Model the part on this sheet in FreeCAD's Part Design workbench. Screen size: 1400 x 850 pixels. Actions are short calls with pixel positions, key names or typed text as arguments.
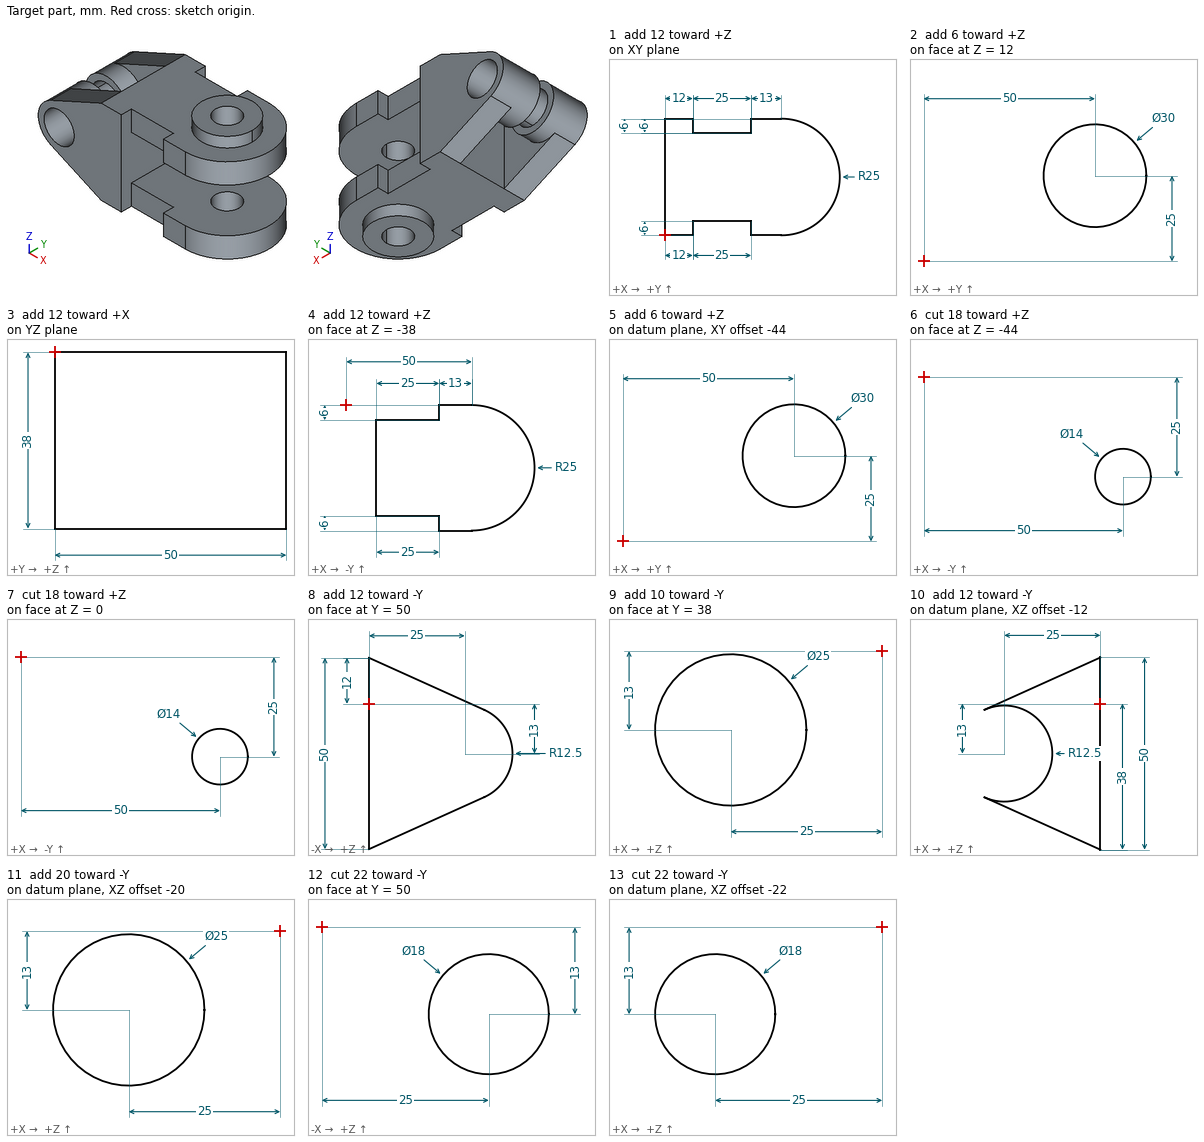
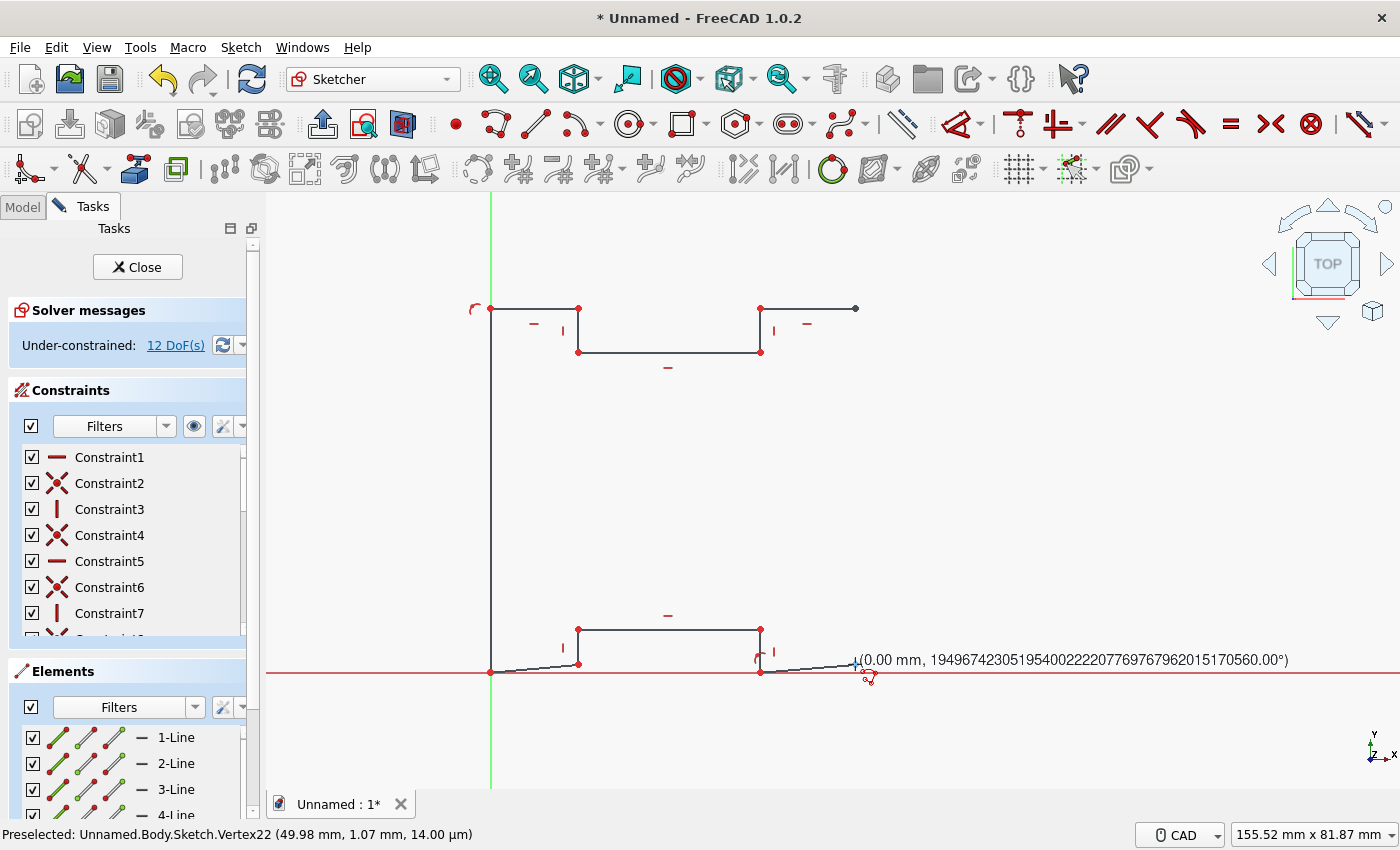
click(602, 124)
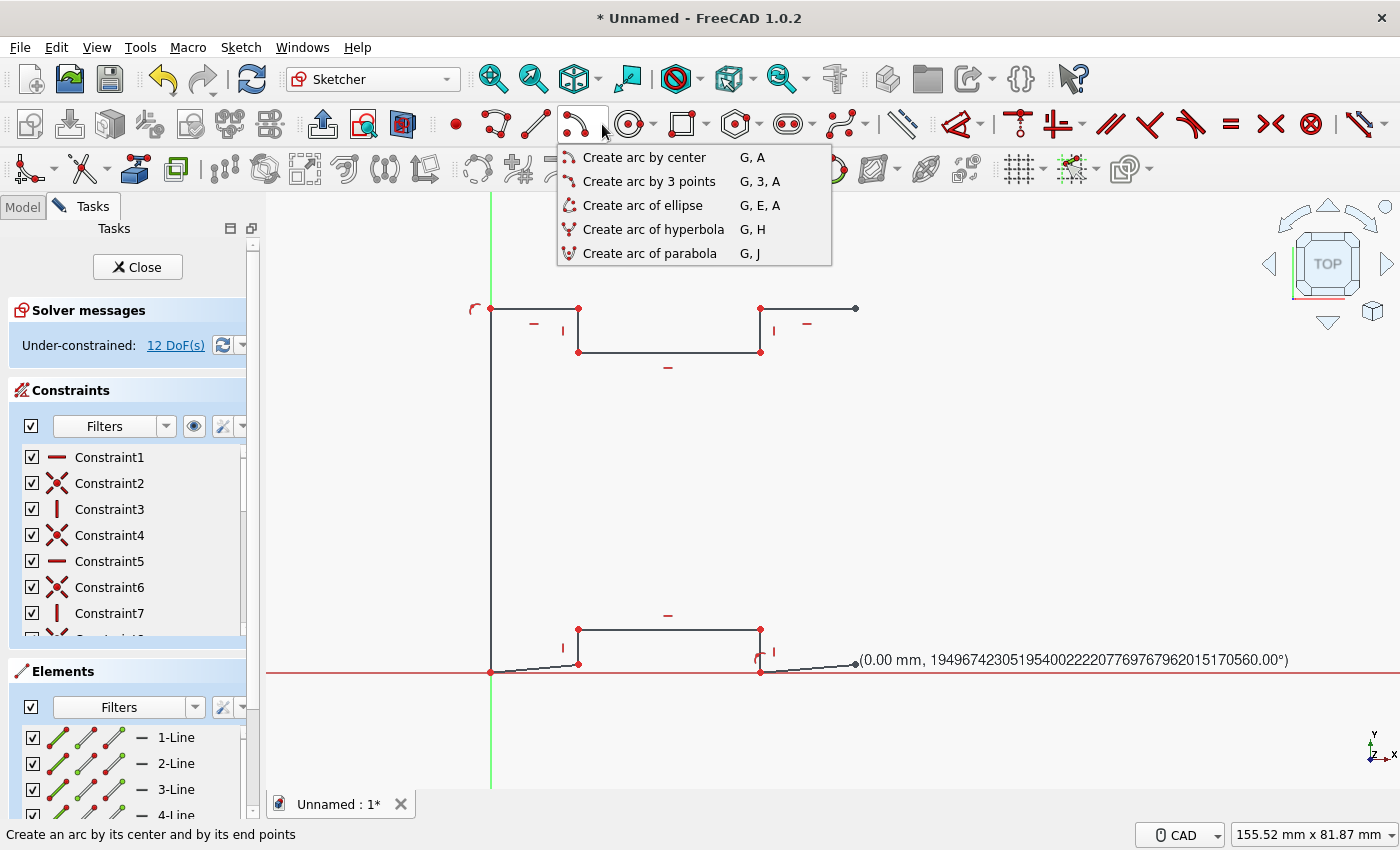
click(694, 181)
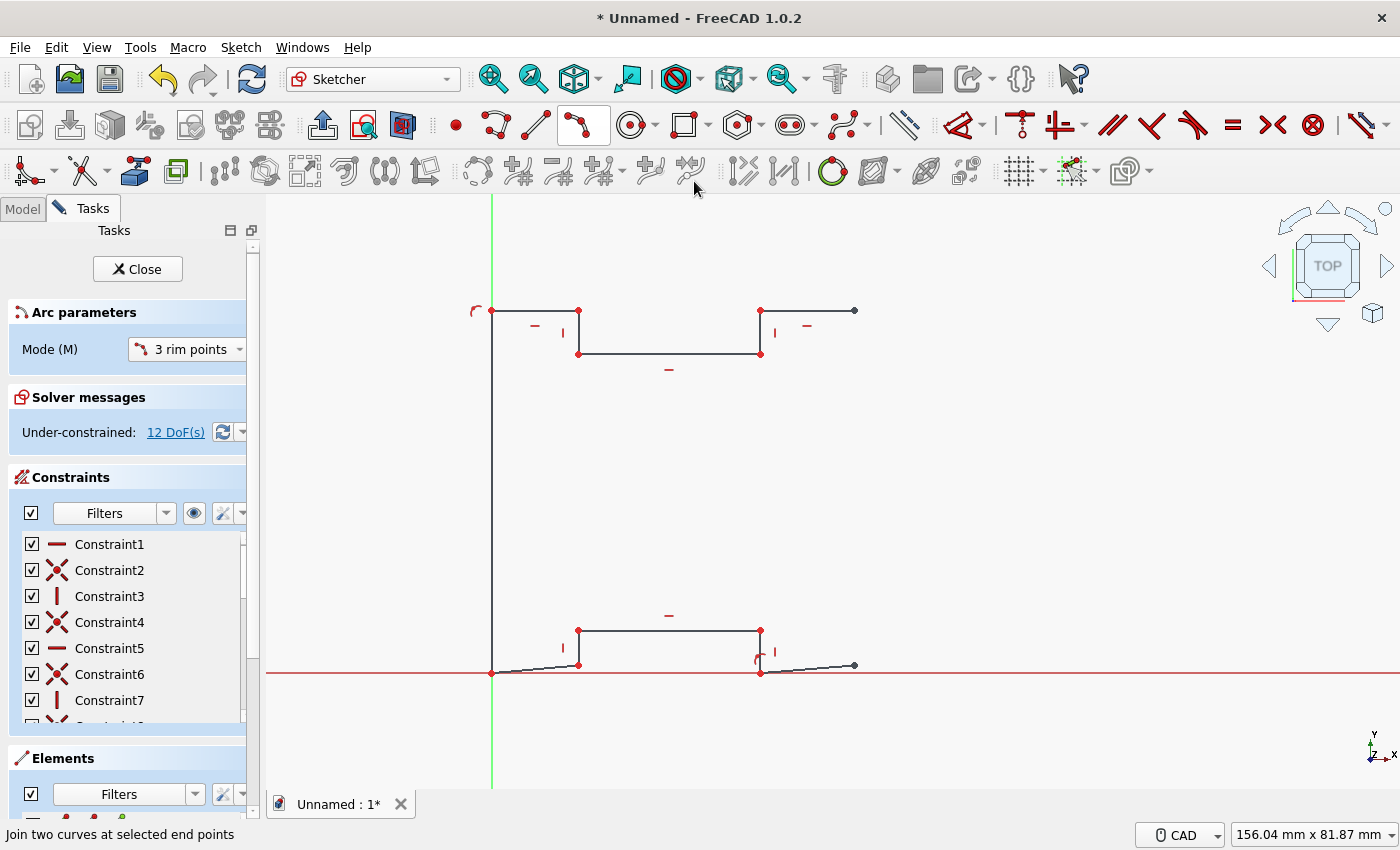
click(855, 665)
click(855, 311)
click(1037, 491)
key(Escape)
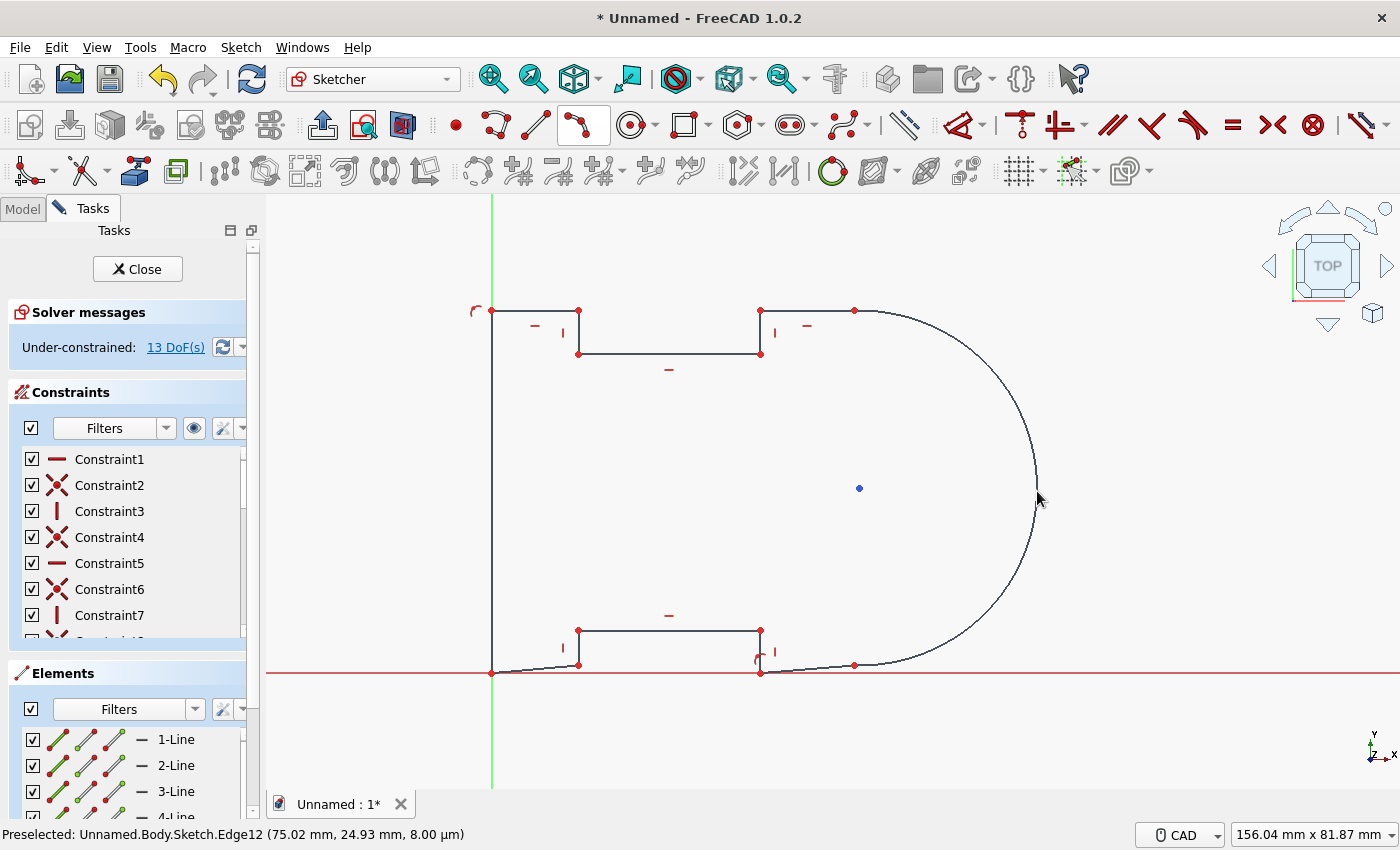
click(827, 311)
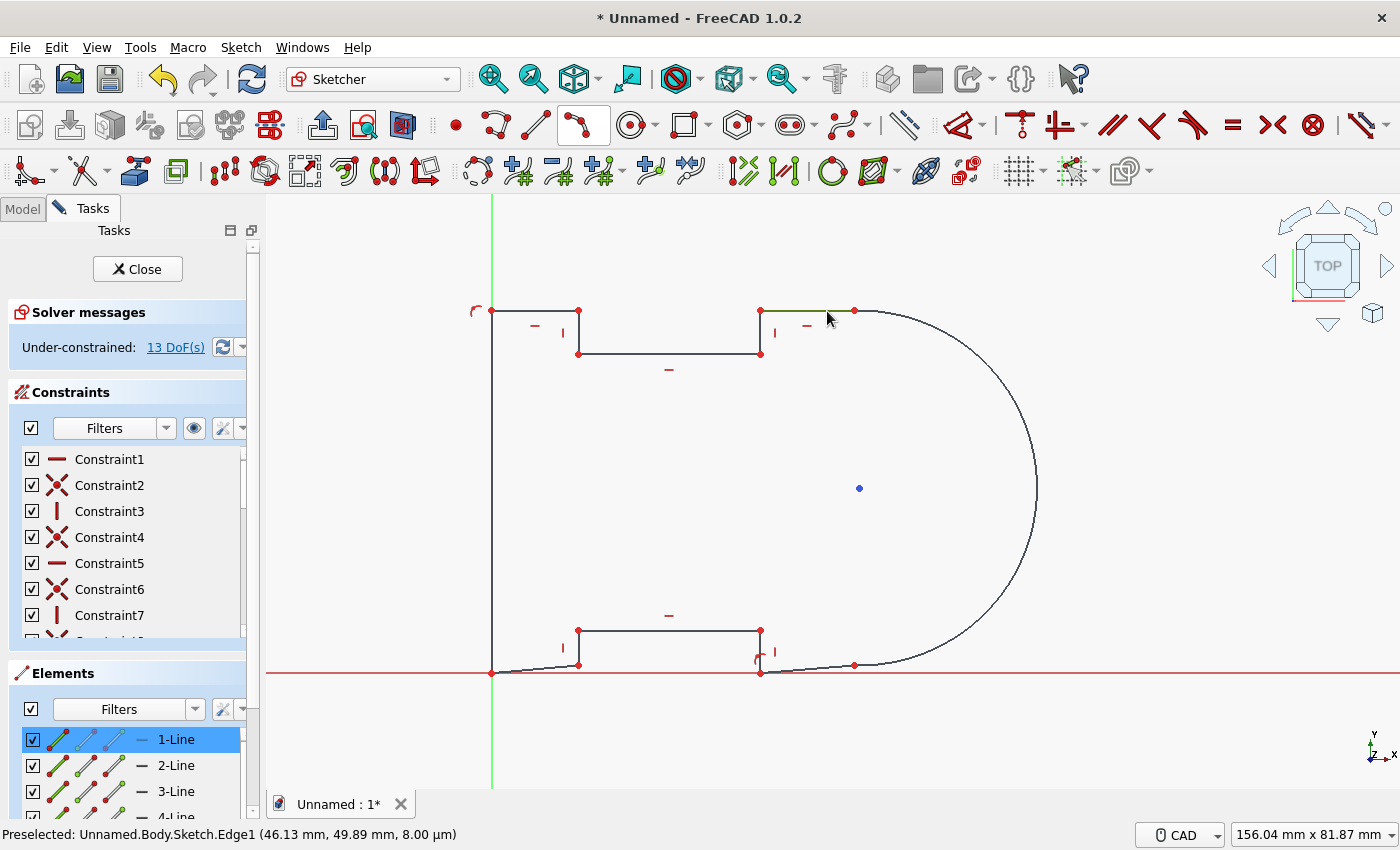
click(1002, 594)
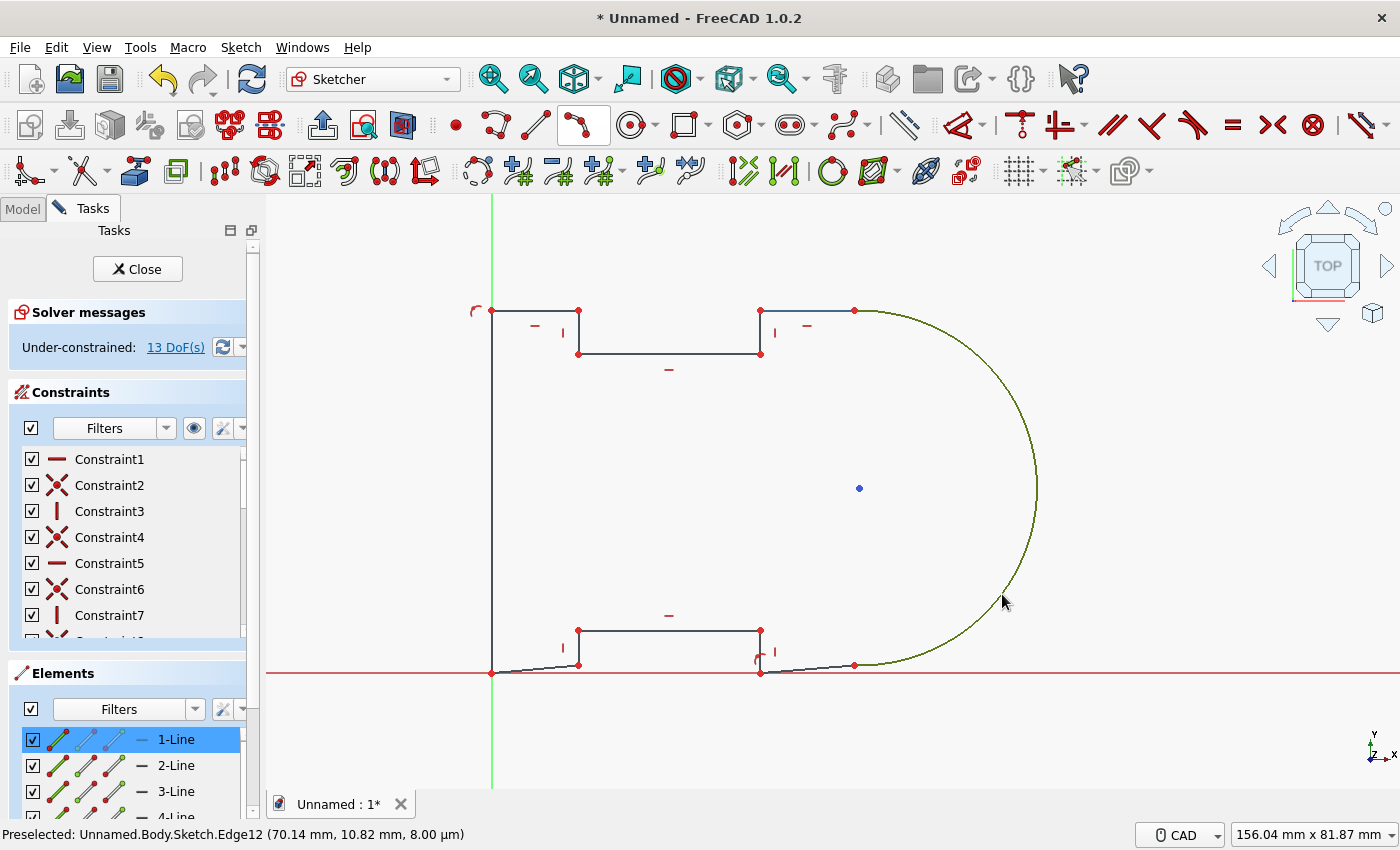
click(1194, 126)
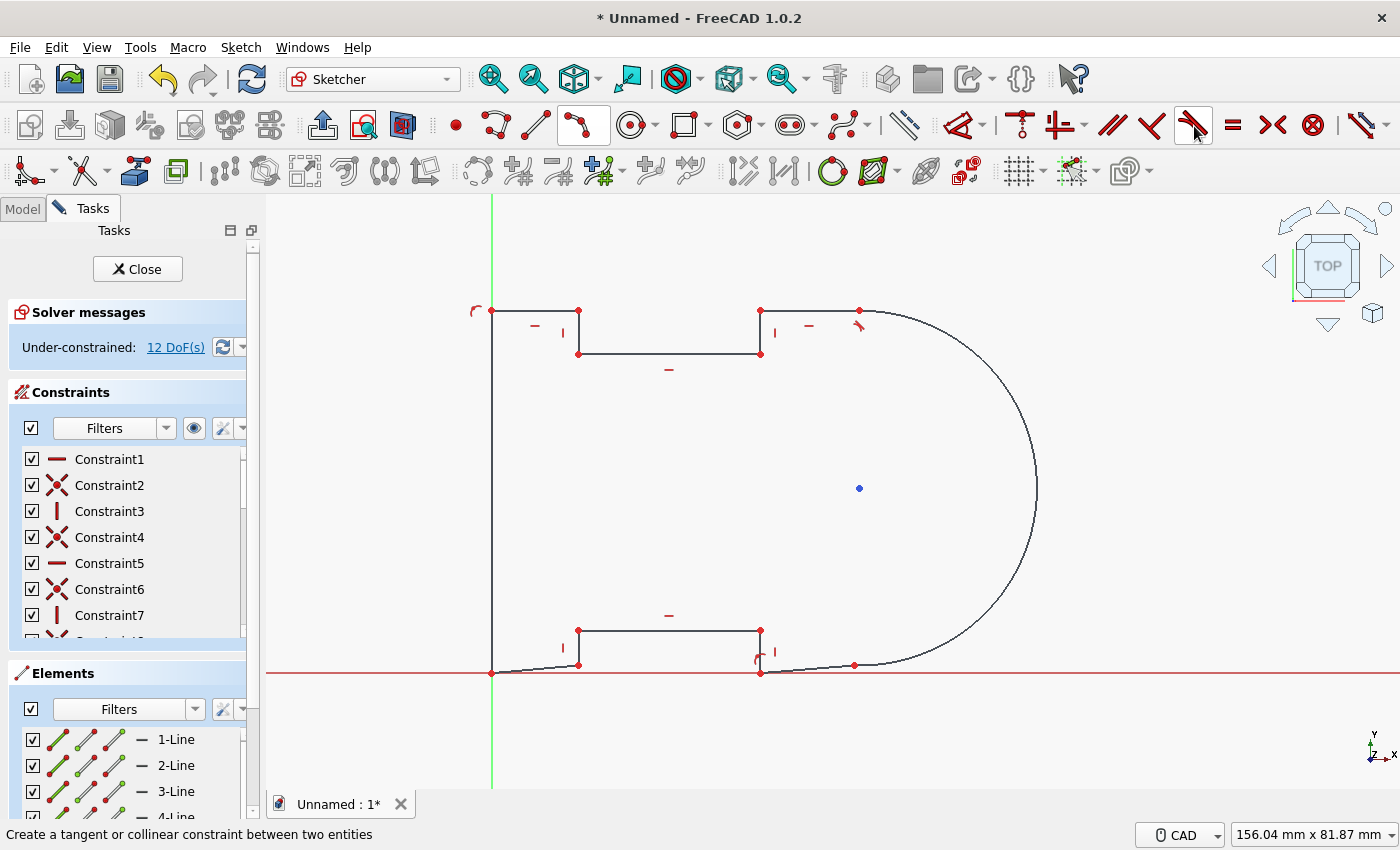
click(789, 671)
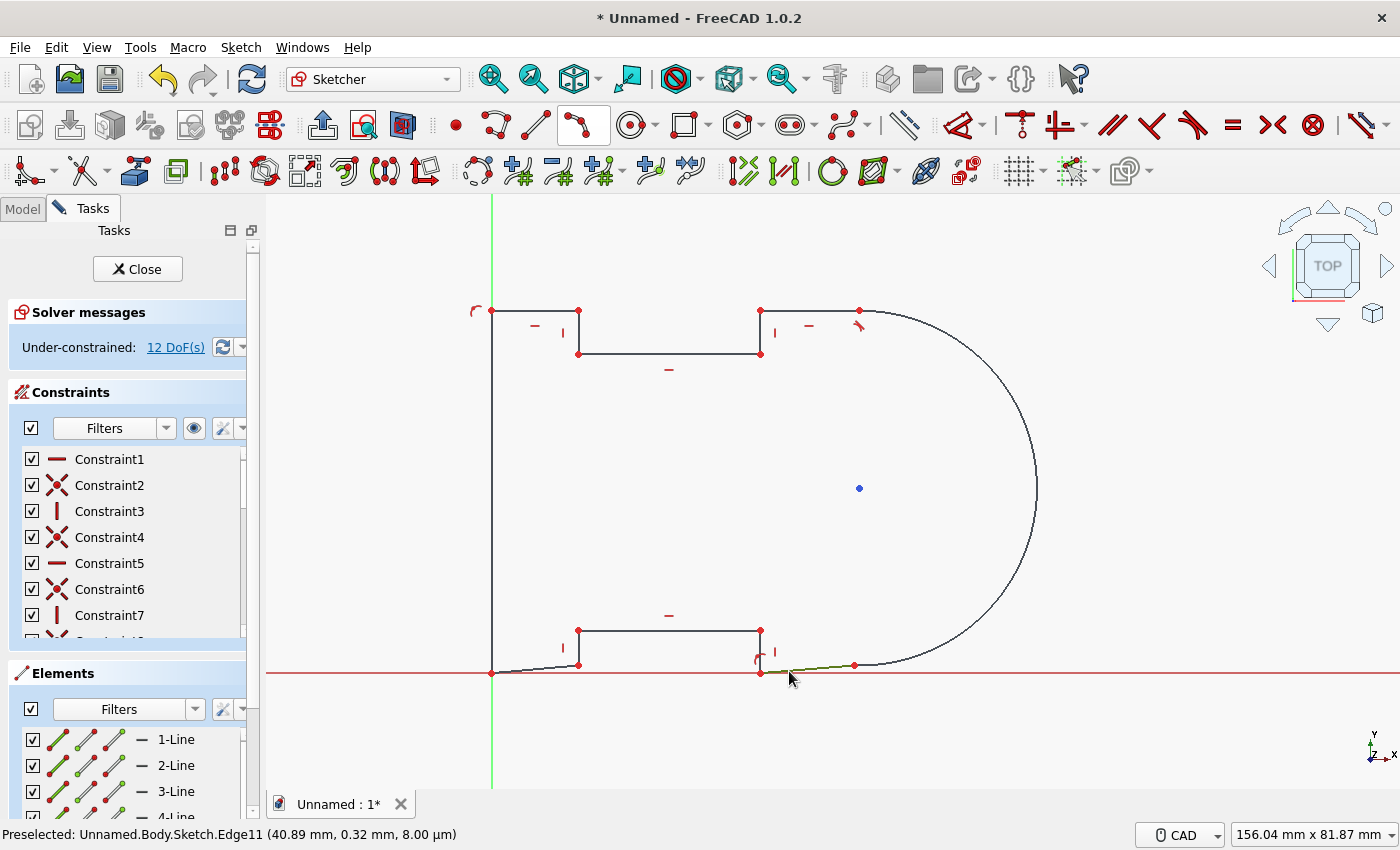
click(1001, 595)